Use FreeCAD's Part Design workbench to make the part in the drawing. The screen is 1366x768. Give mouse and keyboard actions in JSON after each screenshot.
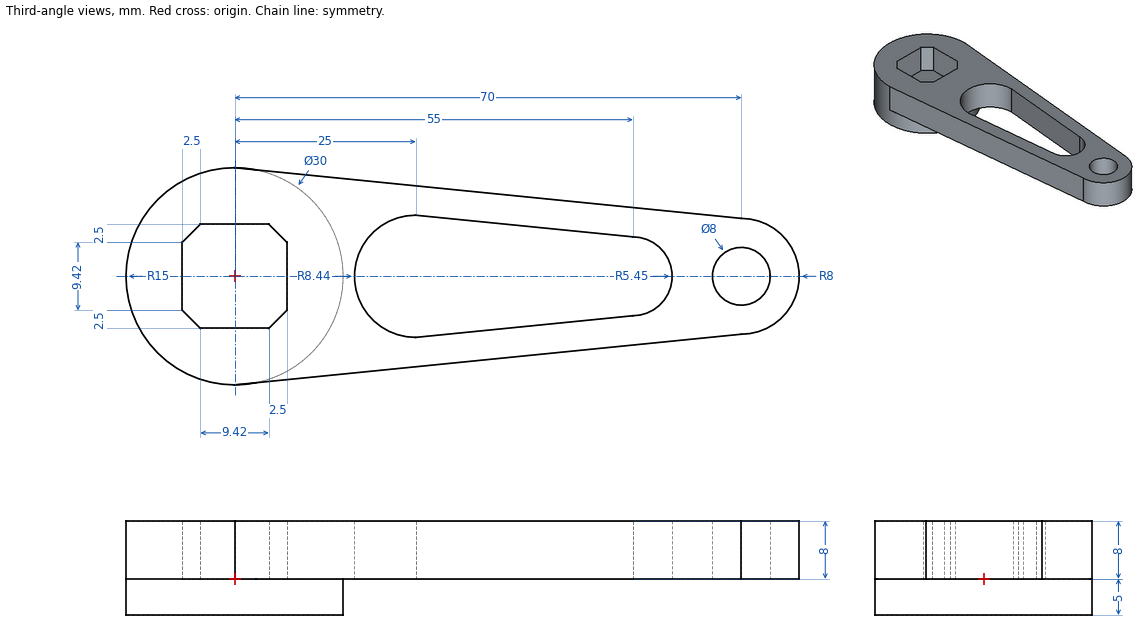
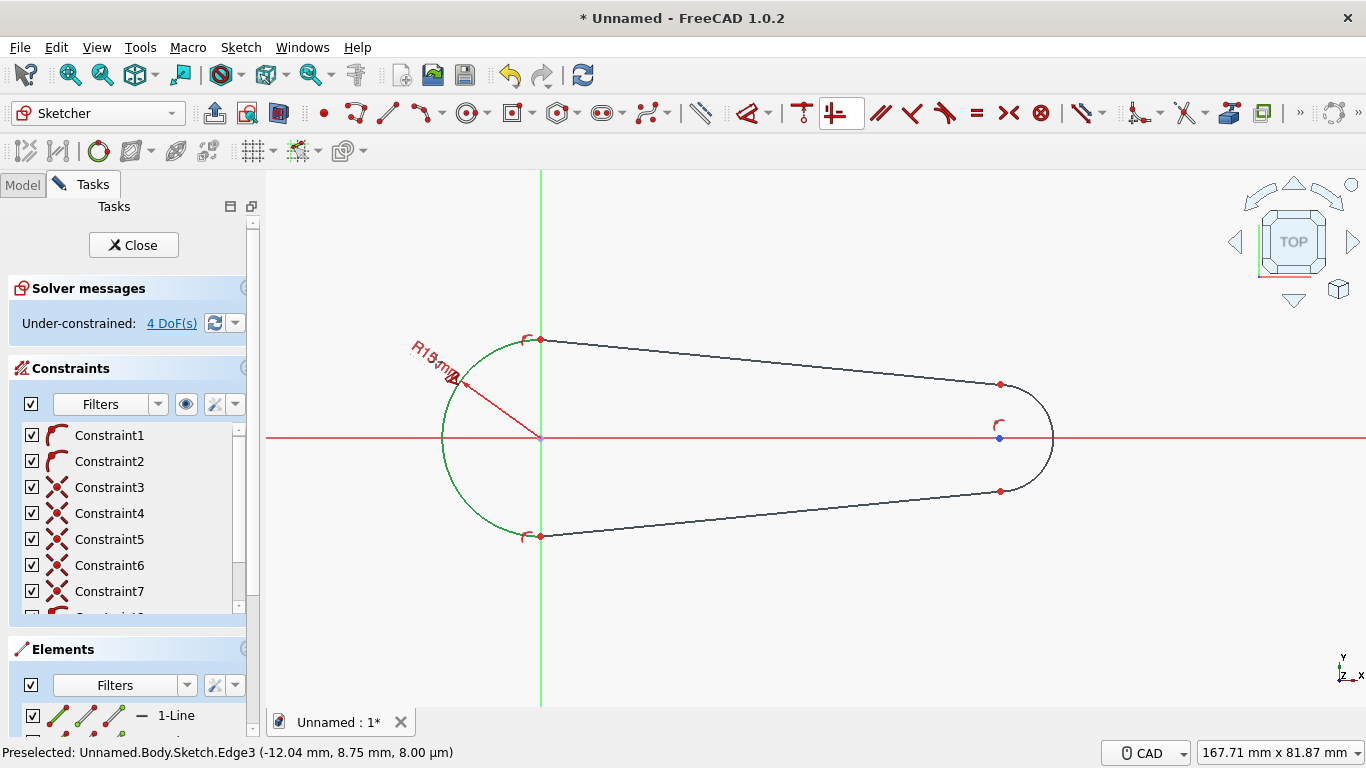
{"action": "left_click", "coordinate": [1043, 470]}
{"action": "left_click", "coordinate": [1069, 489]}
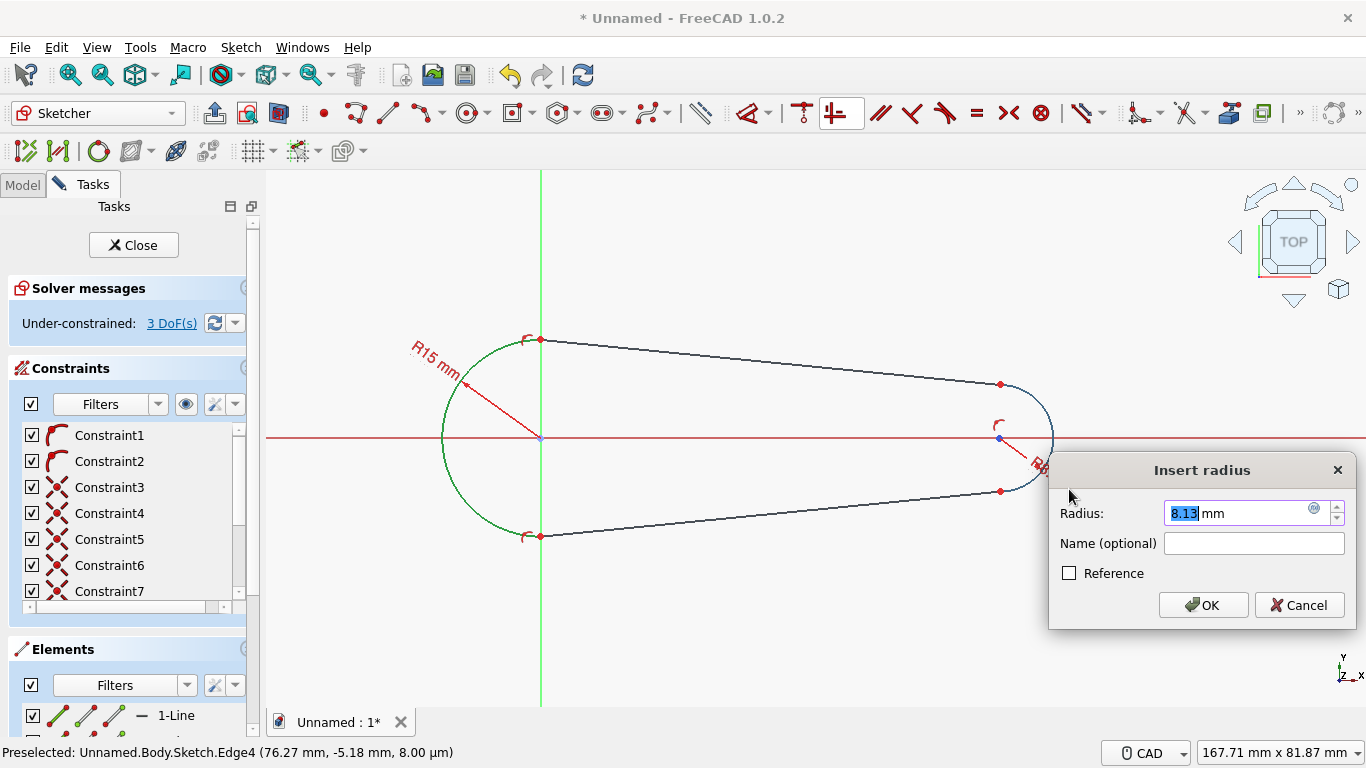
{"action": "type", "text": "8"}
{"action": "key", "text": "Return"}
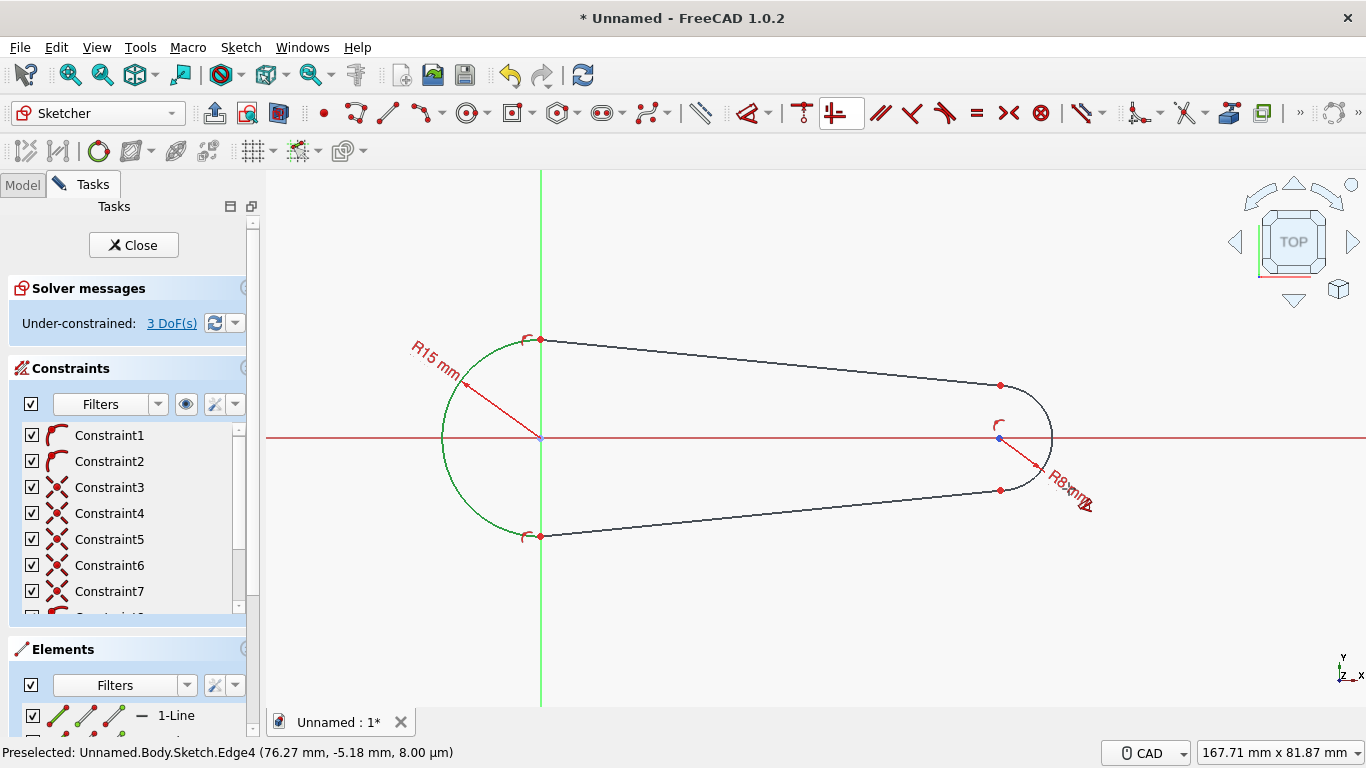
{"action": "left_click", "coordinate": [1000, 386]}
{"action": "left_click", "coordinate": [876, 352]}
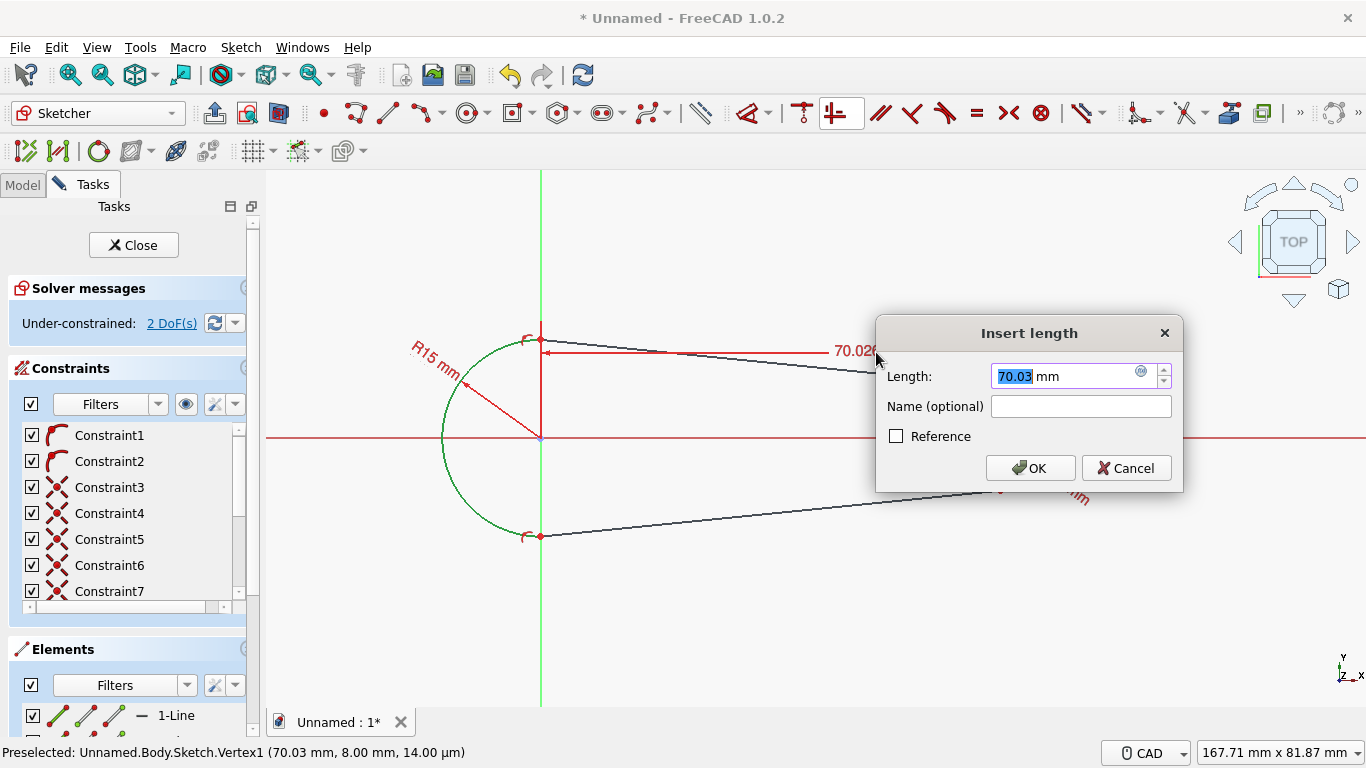
{"action": "type", "text": "70"}
{"action": "key", "text": "Return"}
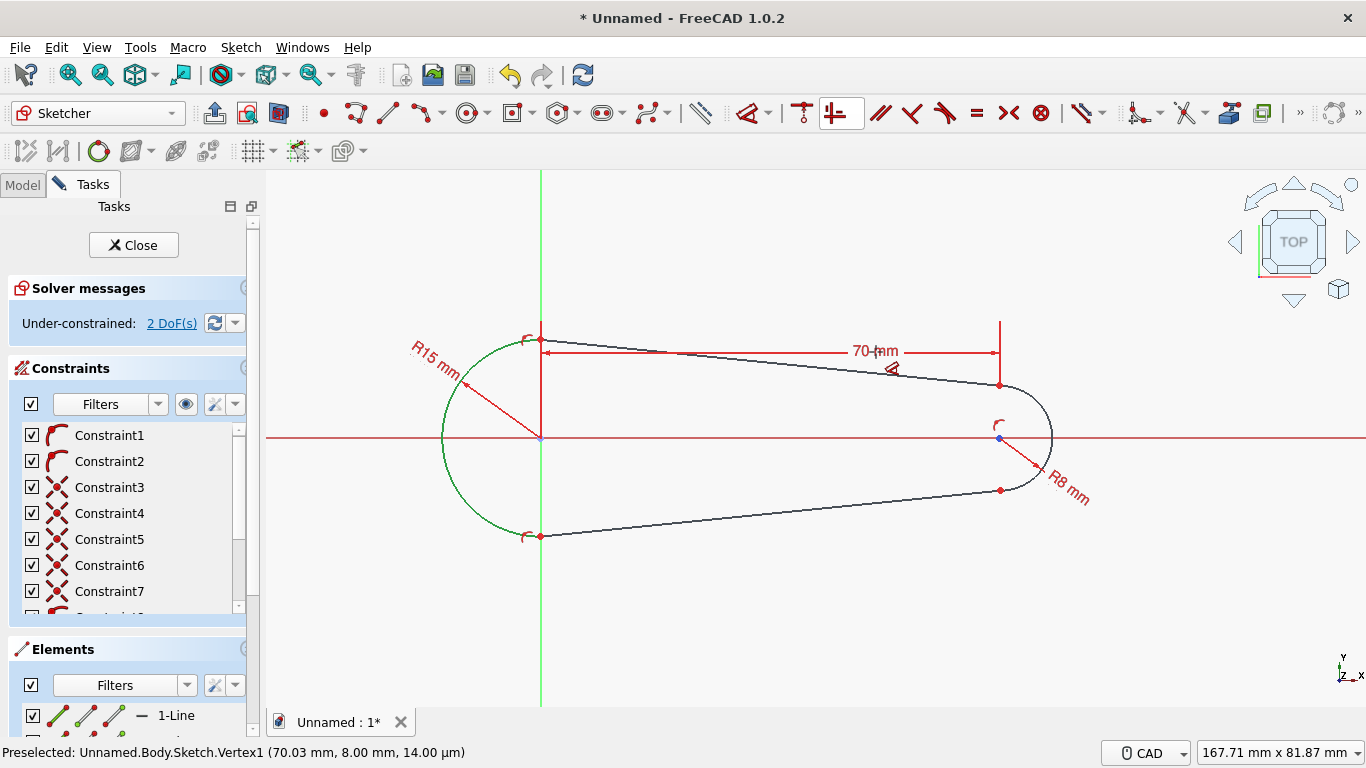
{"action": "left_click", "coordinate": [1000, 491]}
{"action": "left_click", "coordinate": [876, 525]}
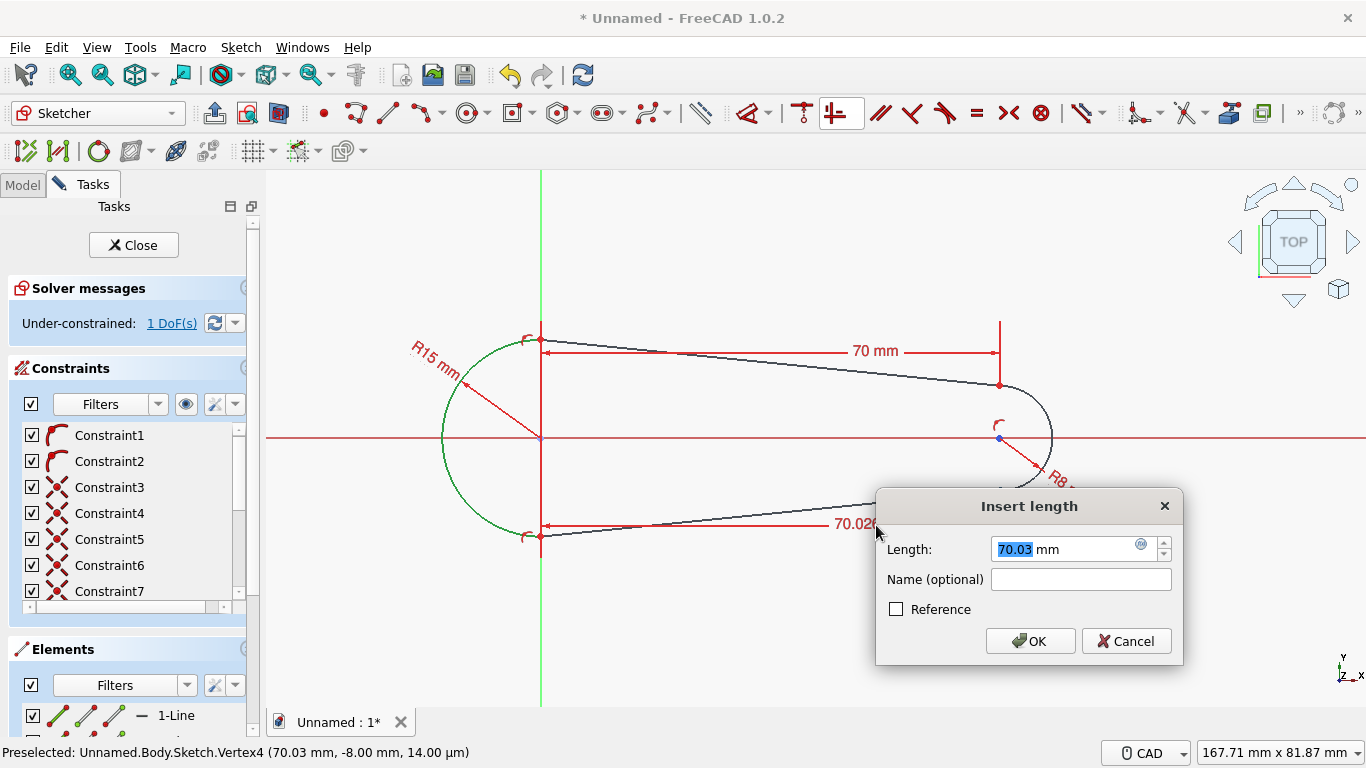
{"action": "type", "text": "70"}
{"action": "key", "text": "Return"}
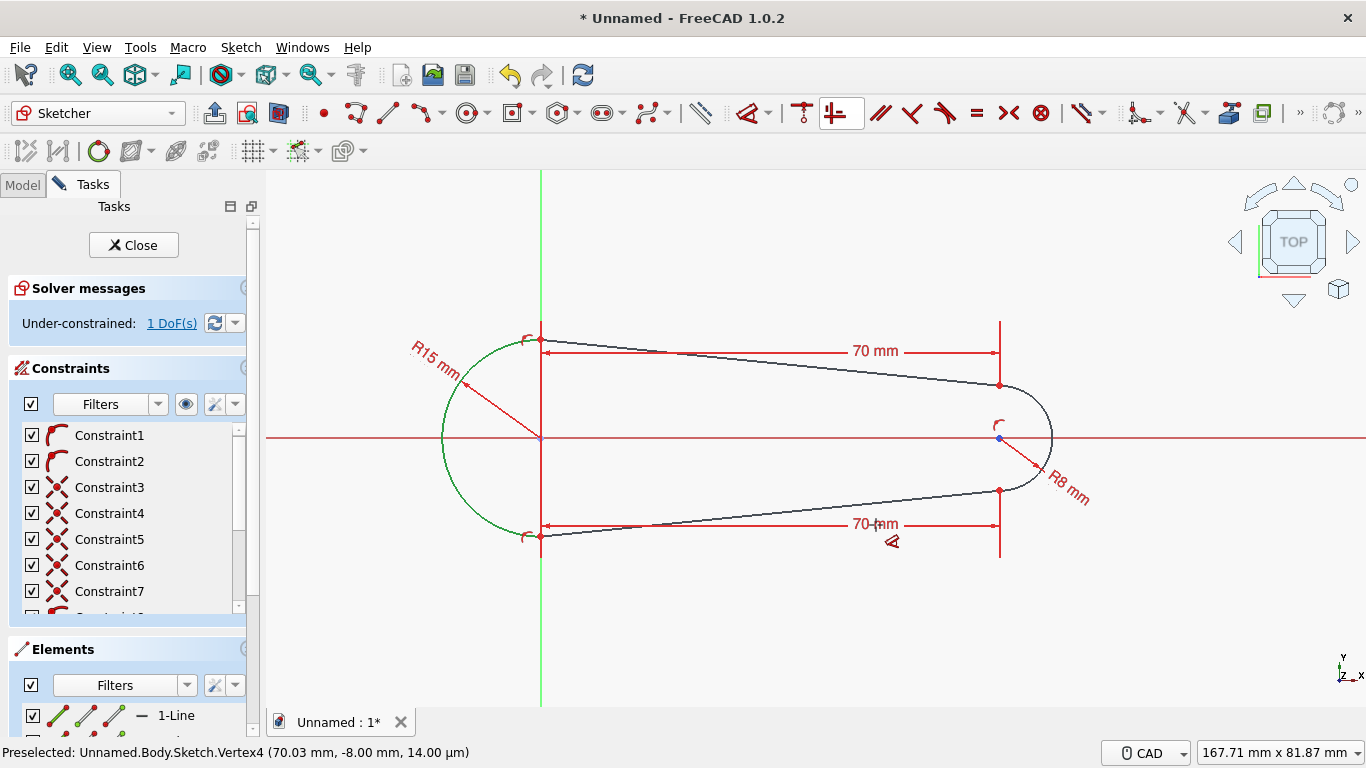
{"action": "left_click", "coordinate": [1000, 438]}
{"action": "left_click", "coordinate": [770, 472]}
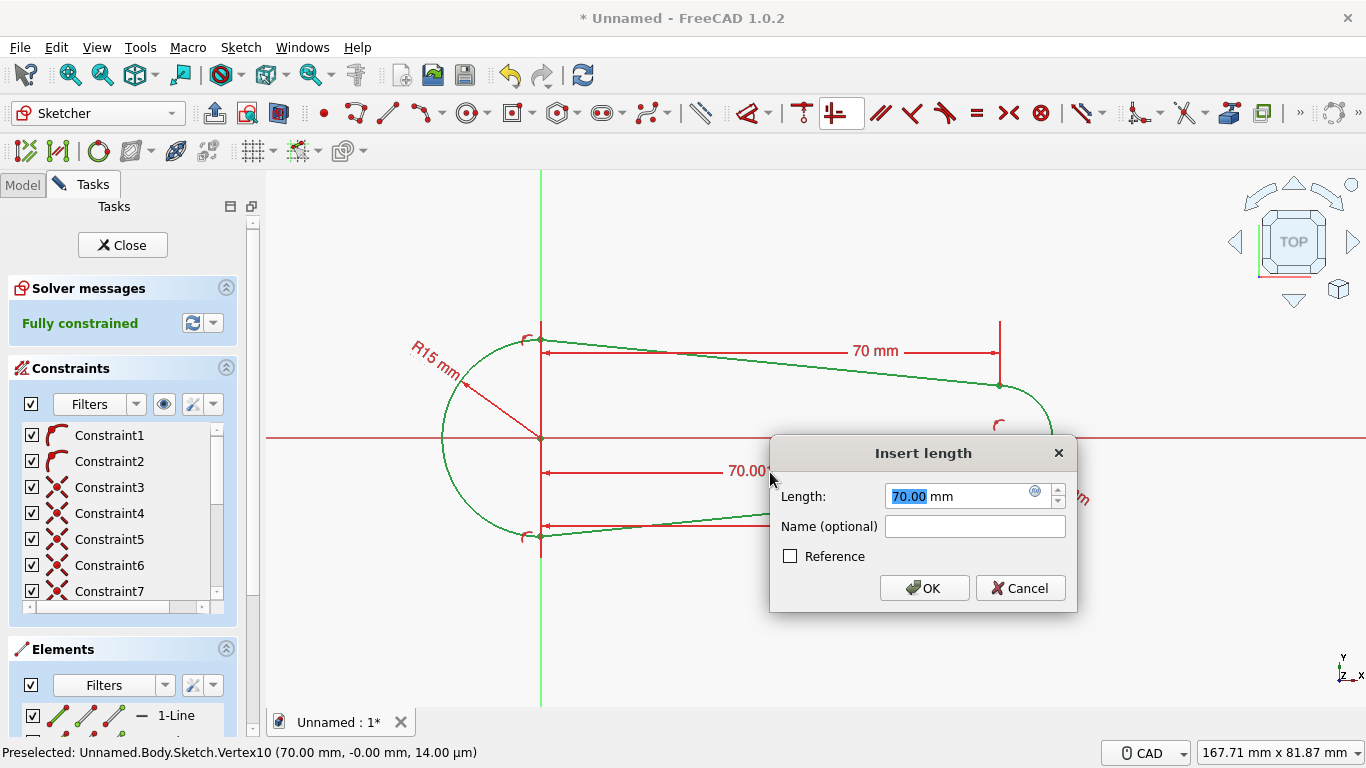
{"action": "type", "text": "70"}
{"action": "key", "text": "Return"}
{"action": "key", "text": "Escape"}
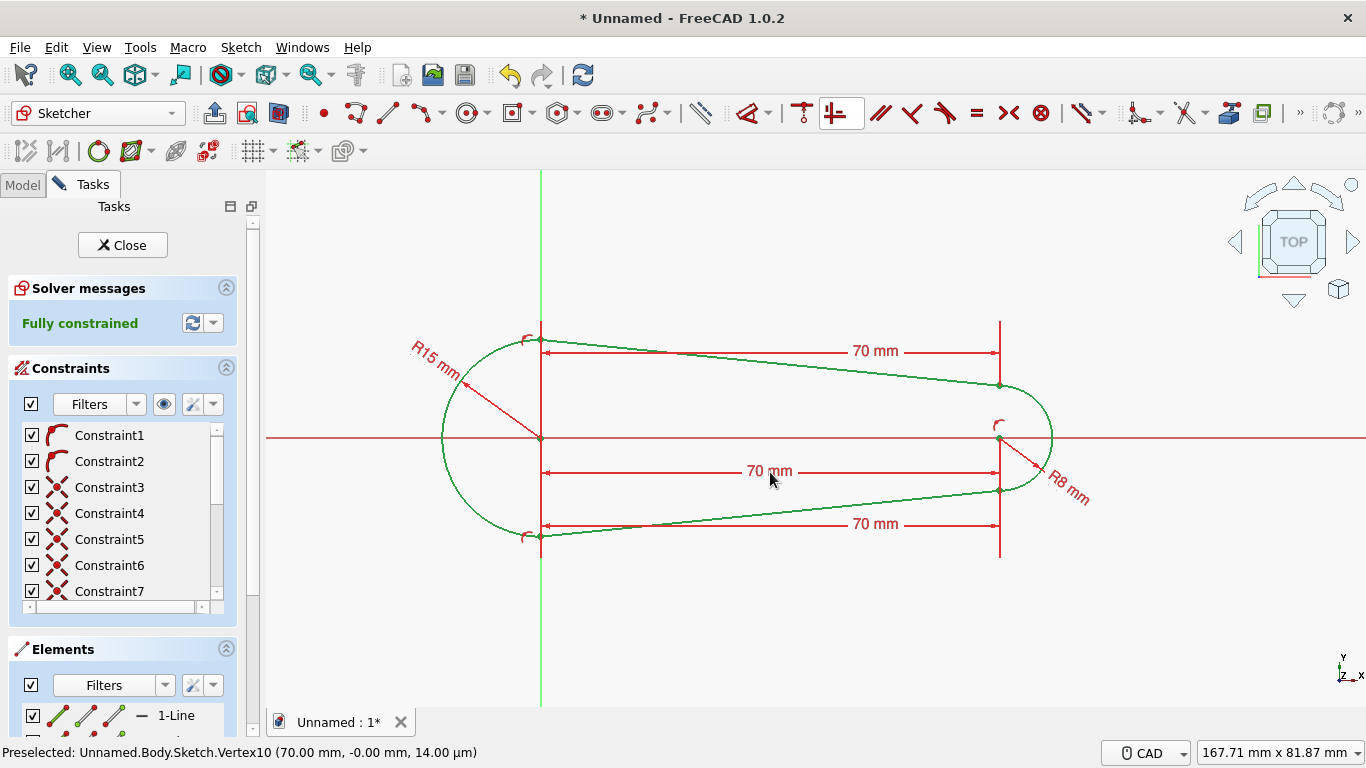
{"action": "left_click", "coordinate": [123, 245]}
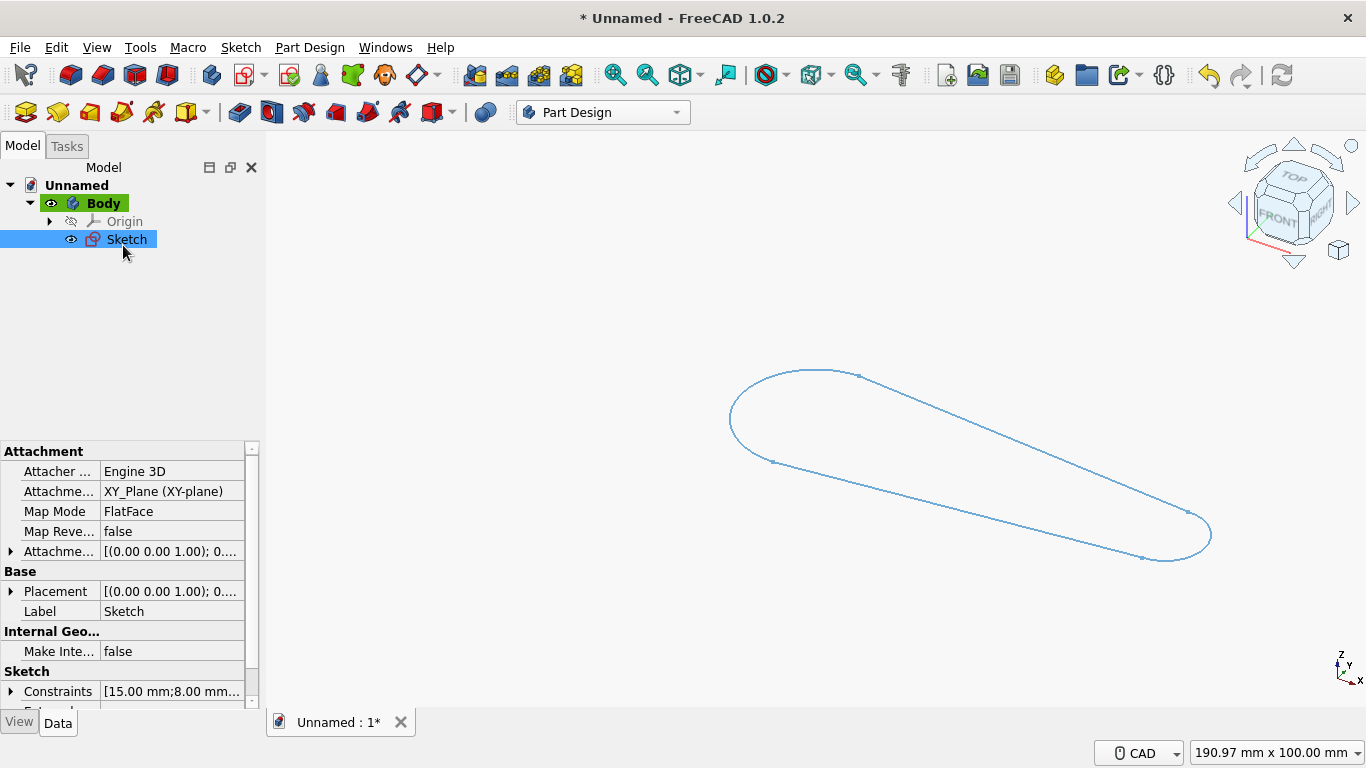
{"action": "left_click", "coordinate": [26, 112]}